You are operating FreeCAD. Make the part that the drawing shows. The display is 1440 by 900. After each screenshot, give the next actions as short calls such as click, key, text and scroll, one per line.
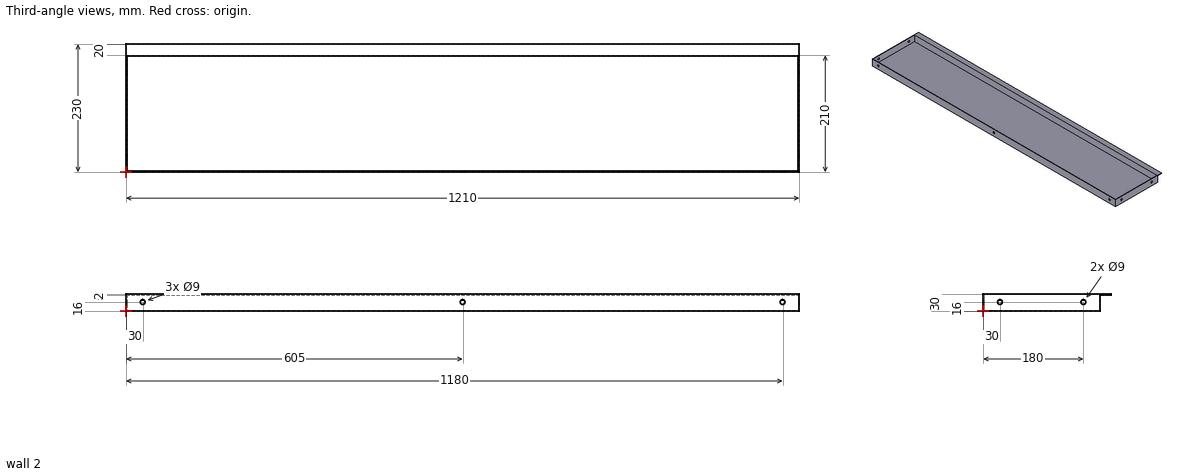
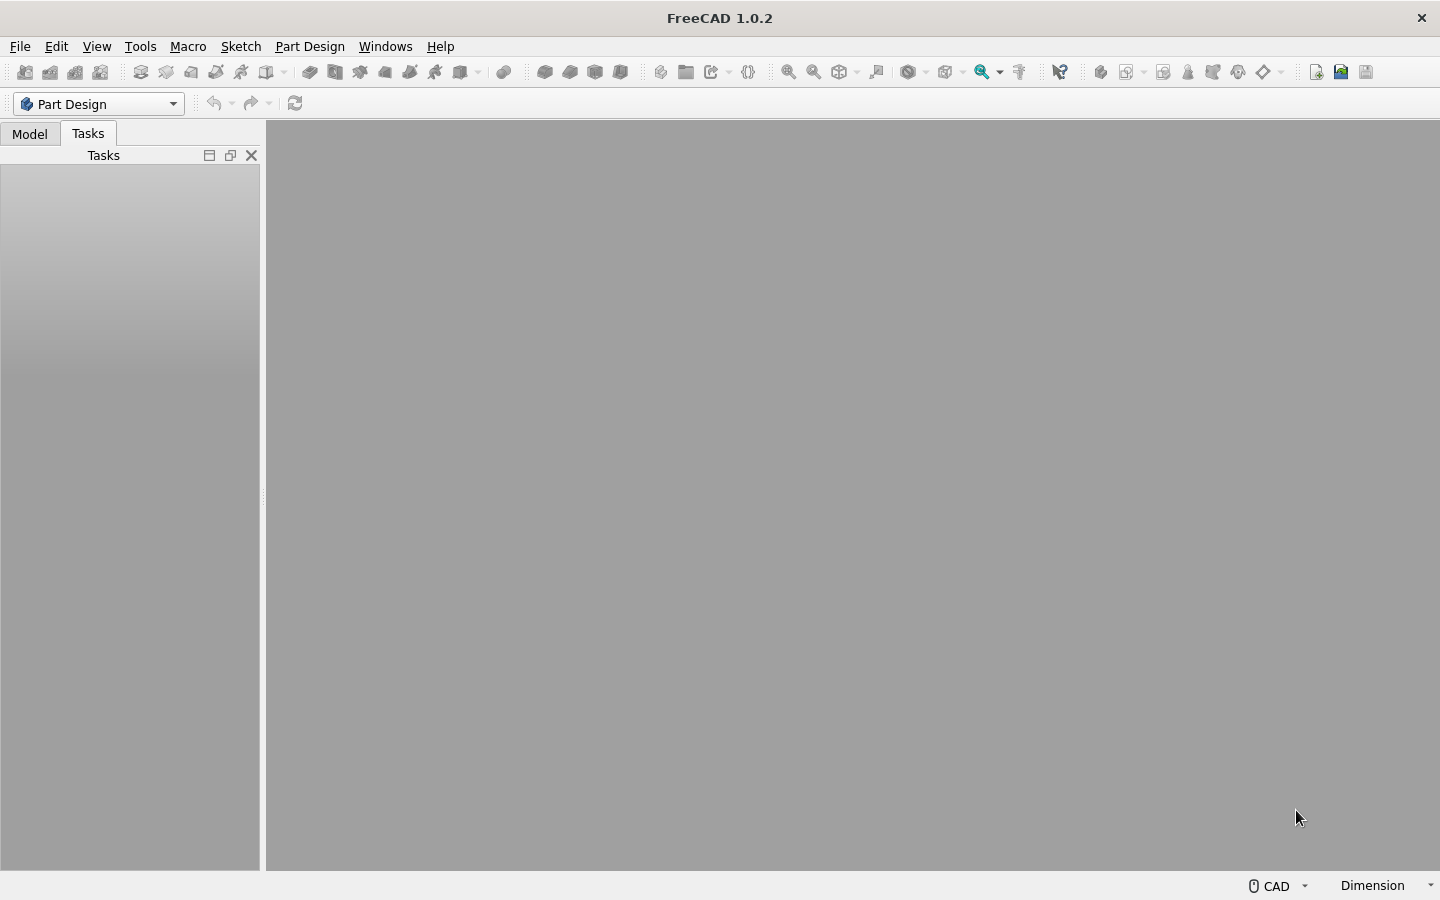
key(ctrl+n)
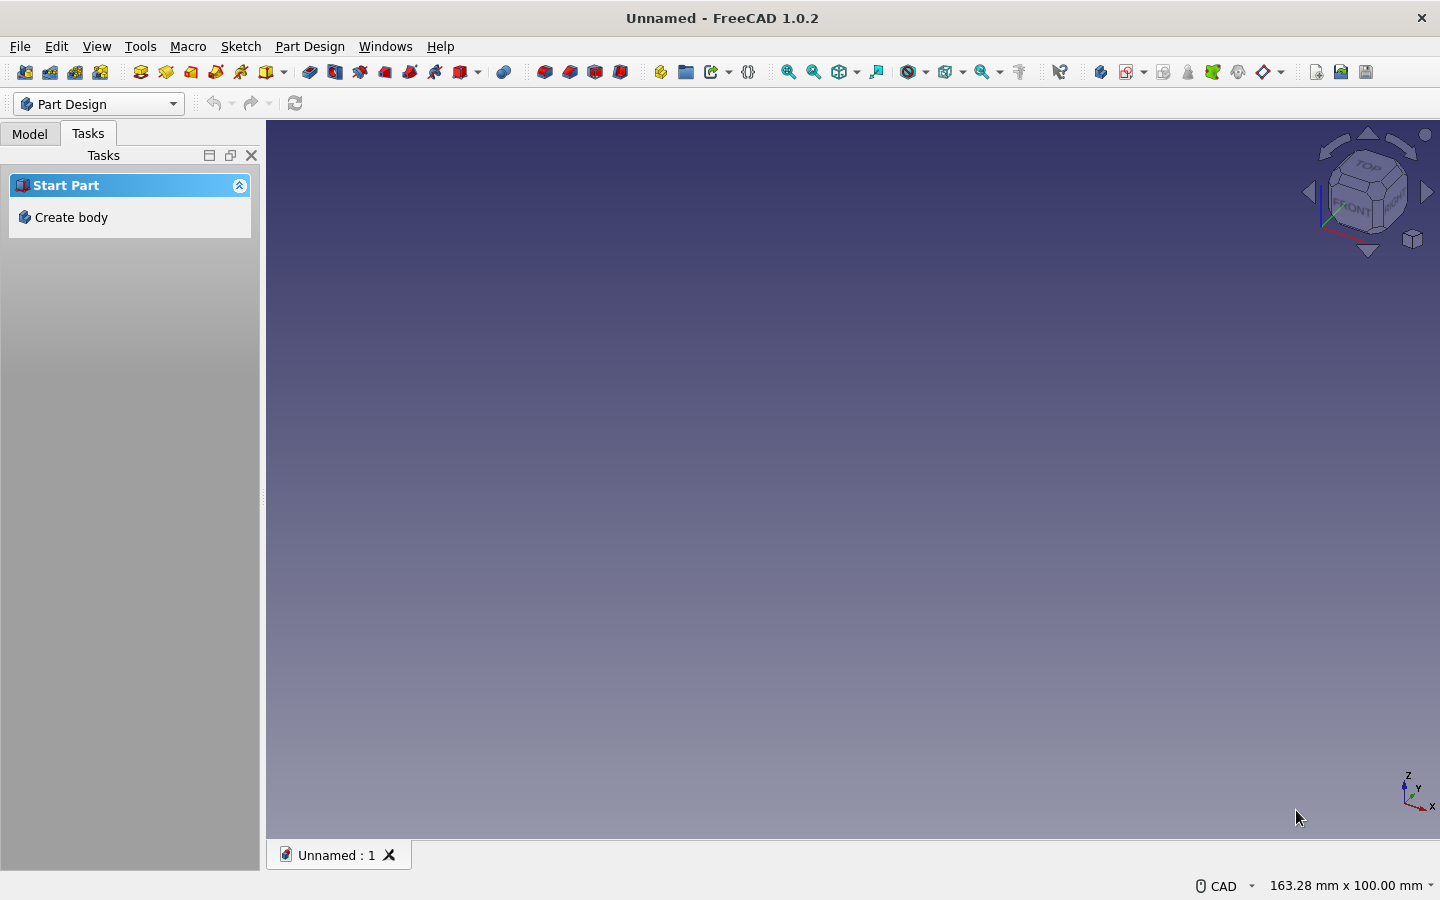
click(1126, 72)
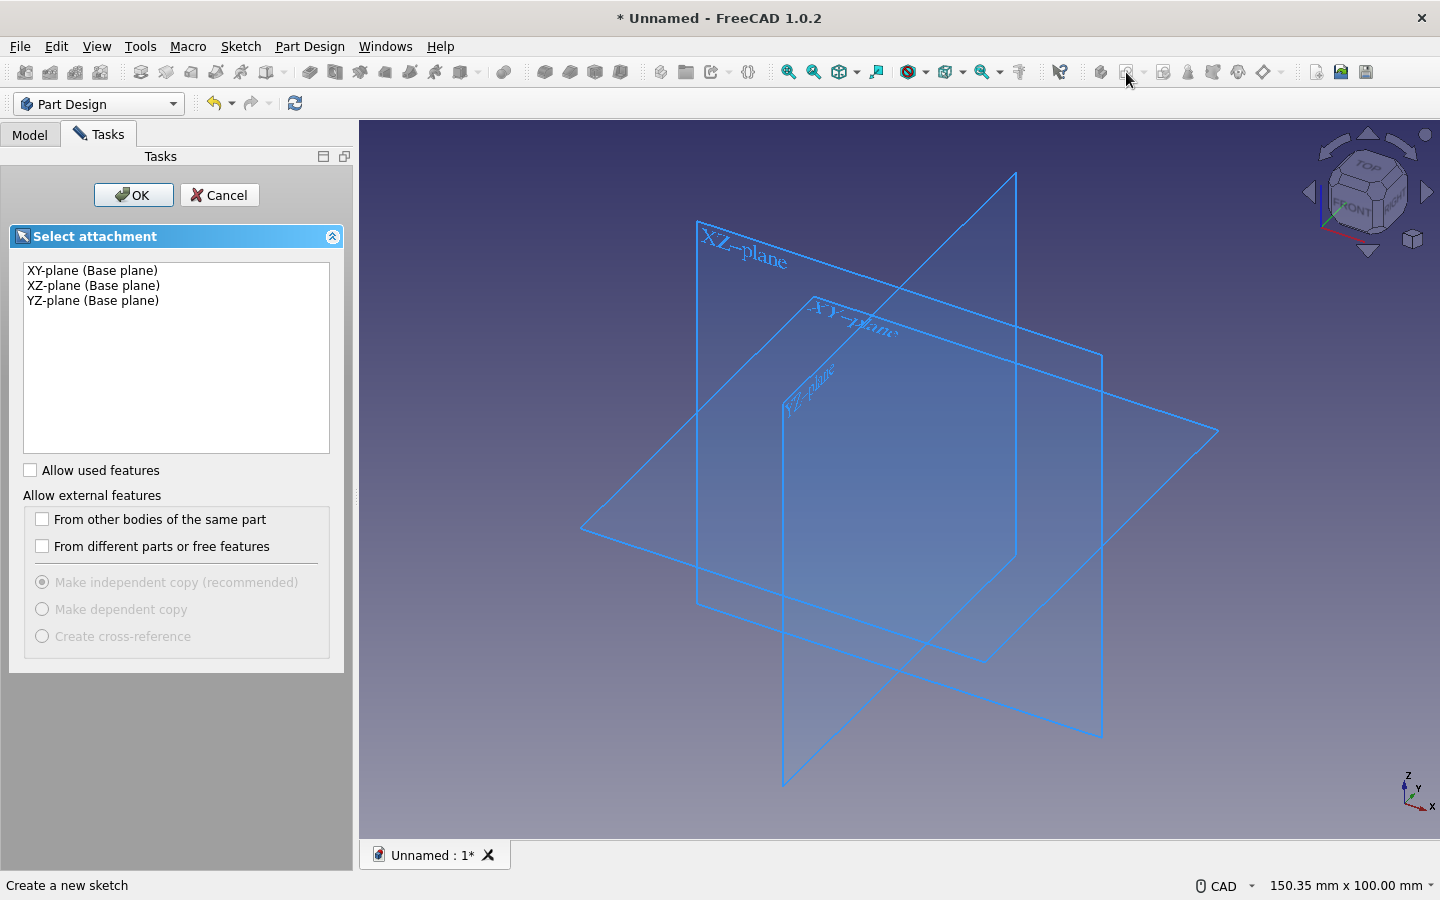
click(84, 270)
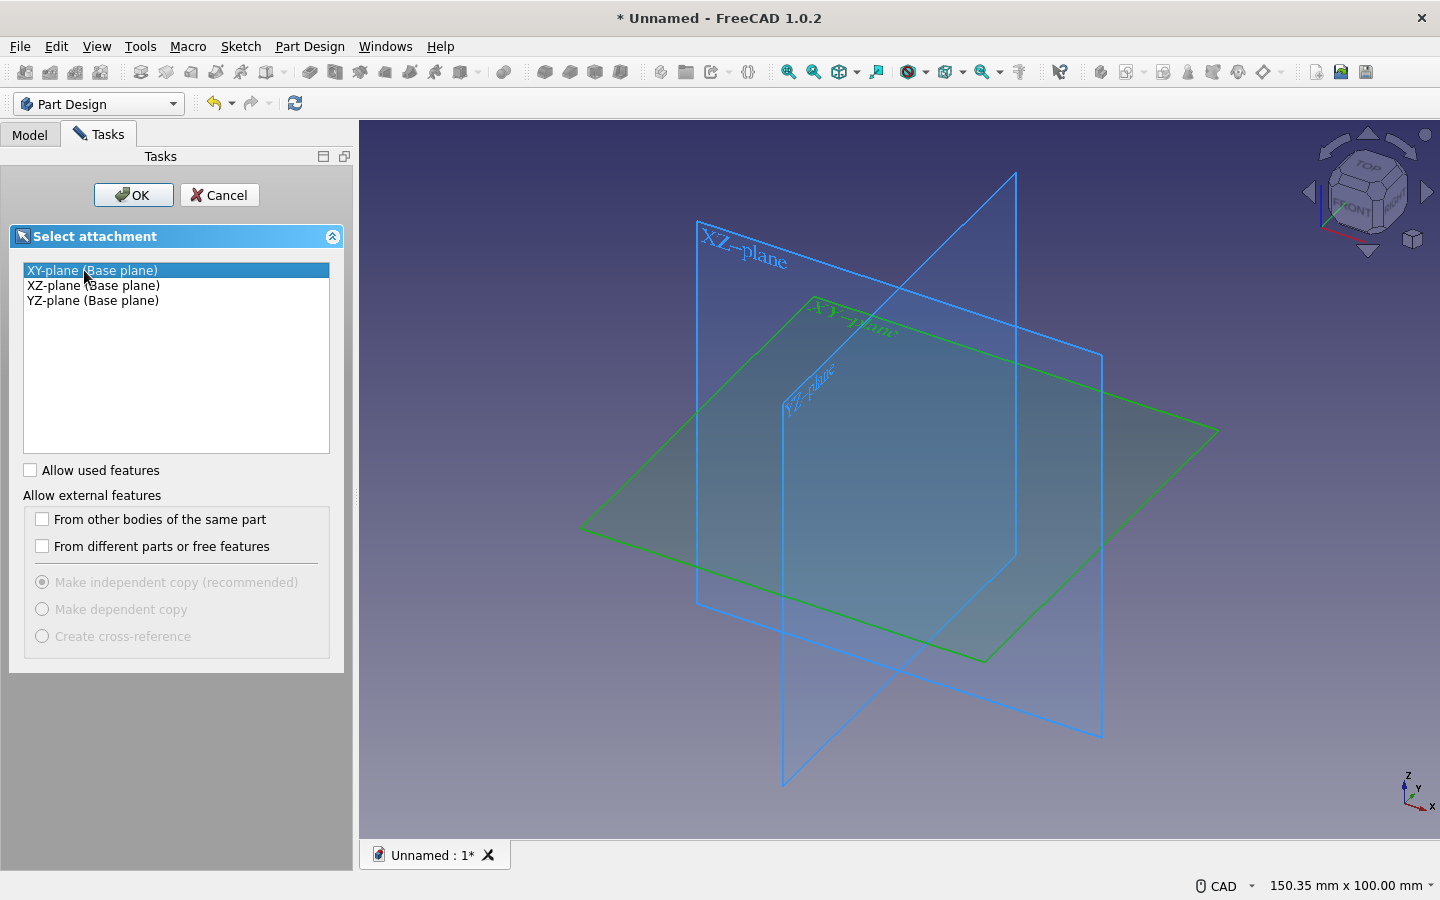
click(134, 195)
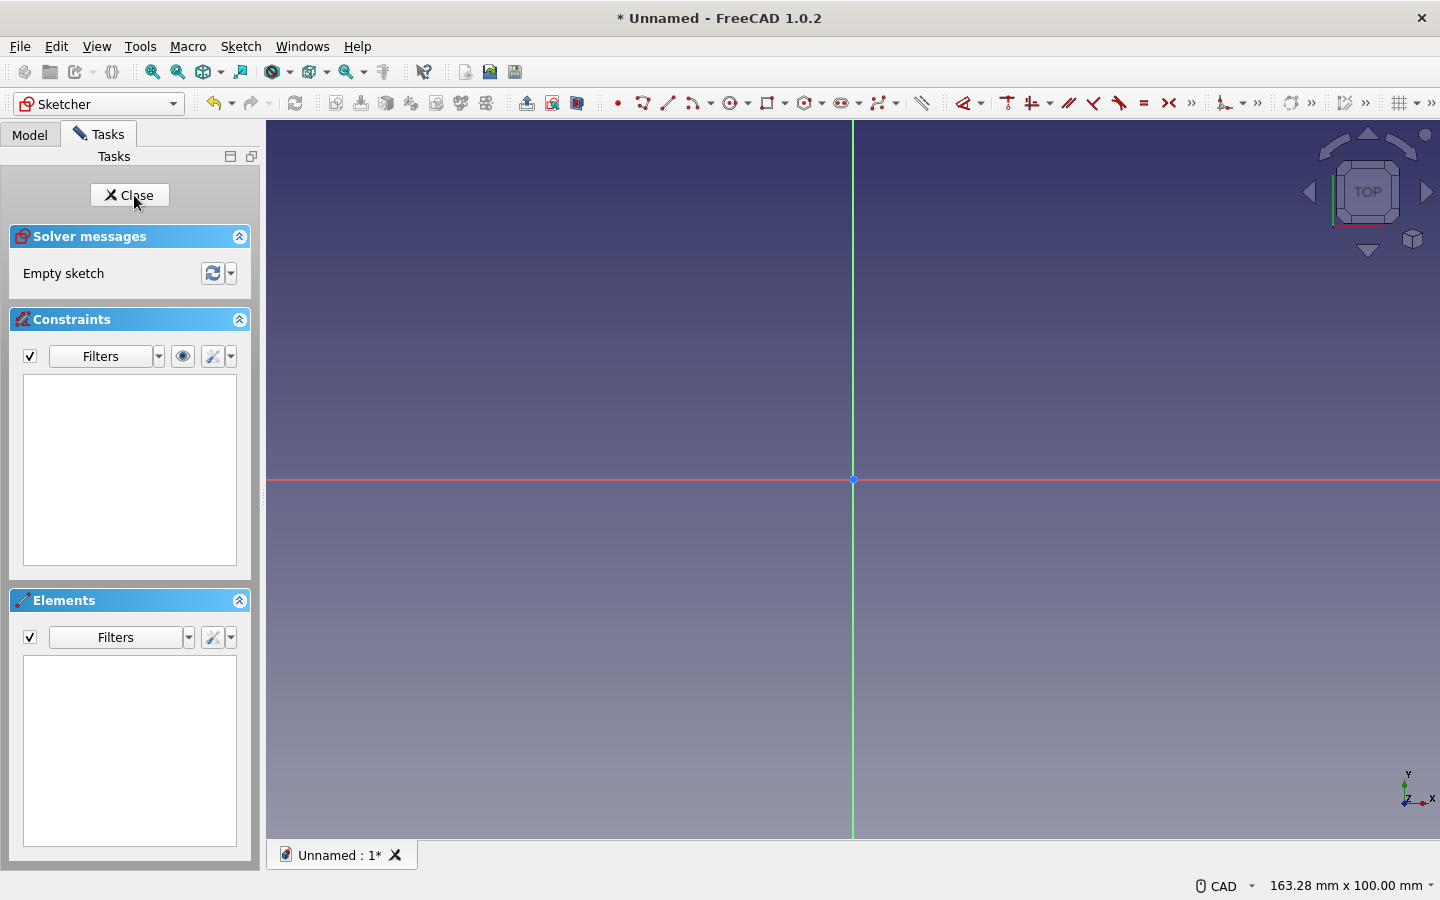
scroll(430, 540, down, 13)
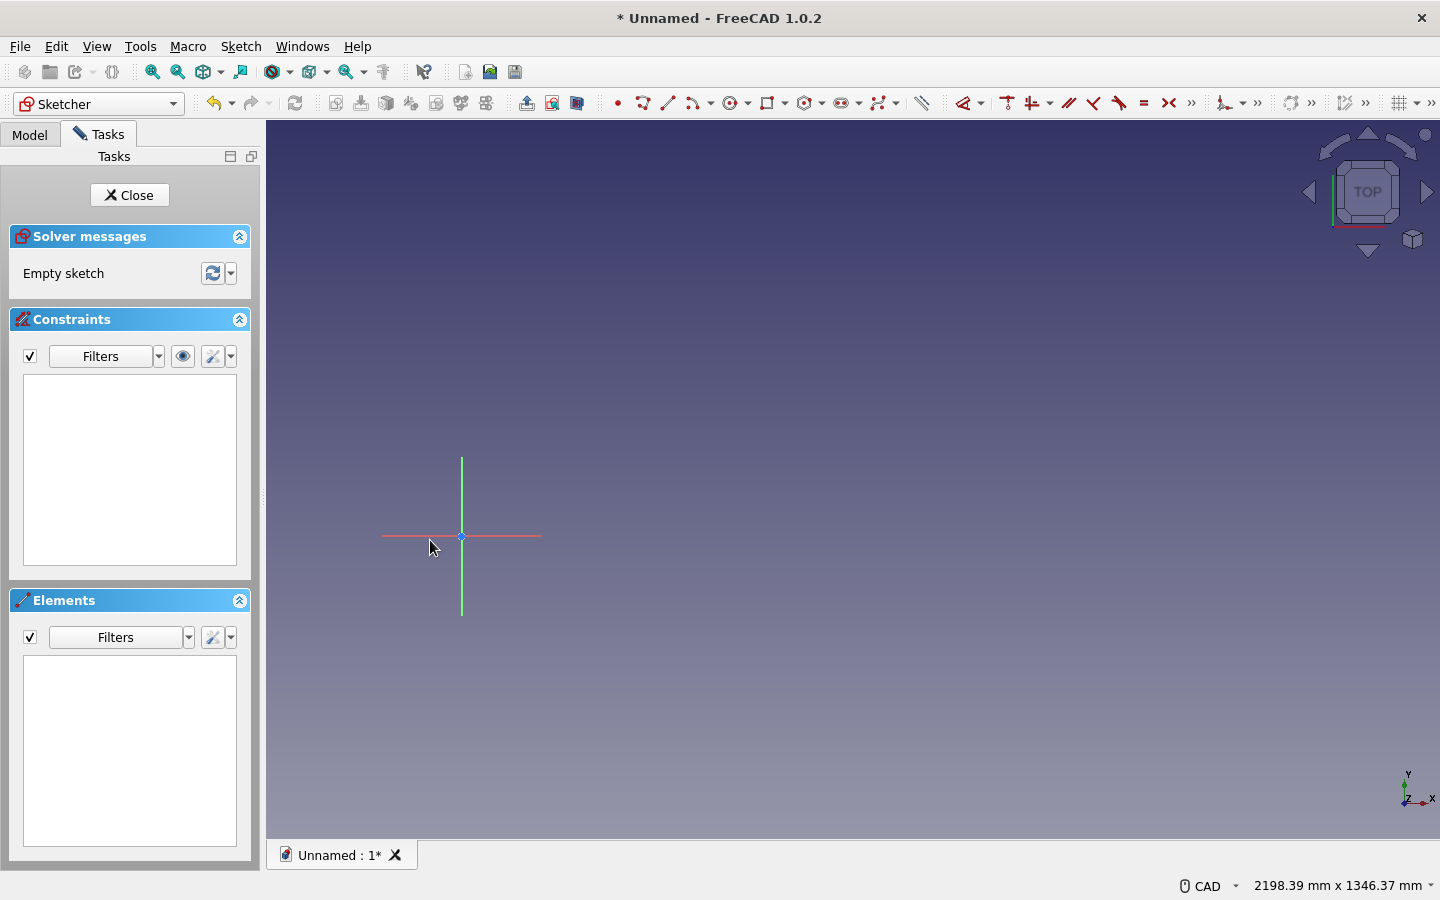
click(766, 104)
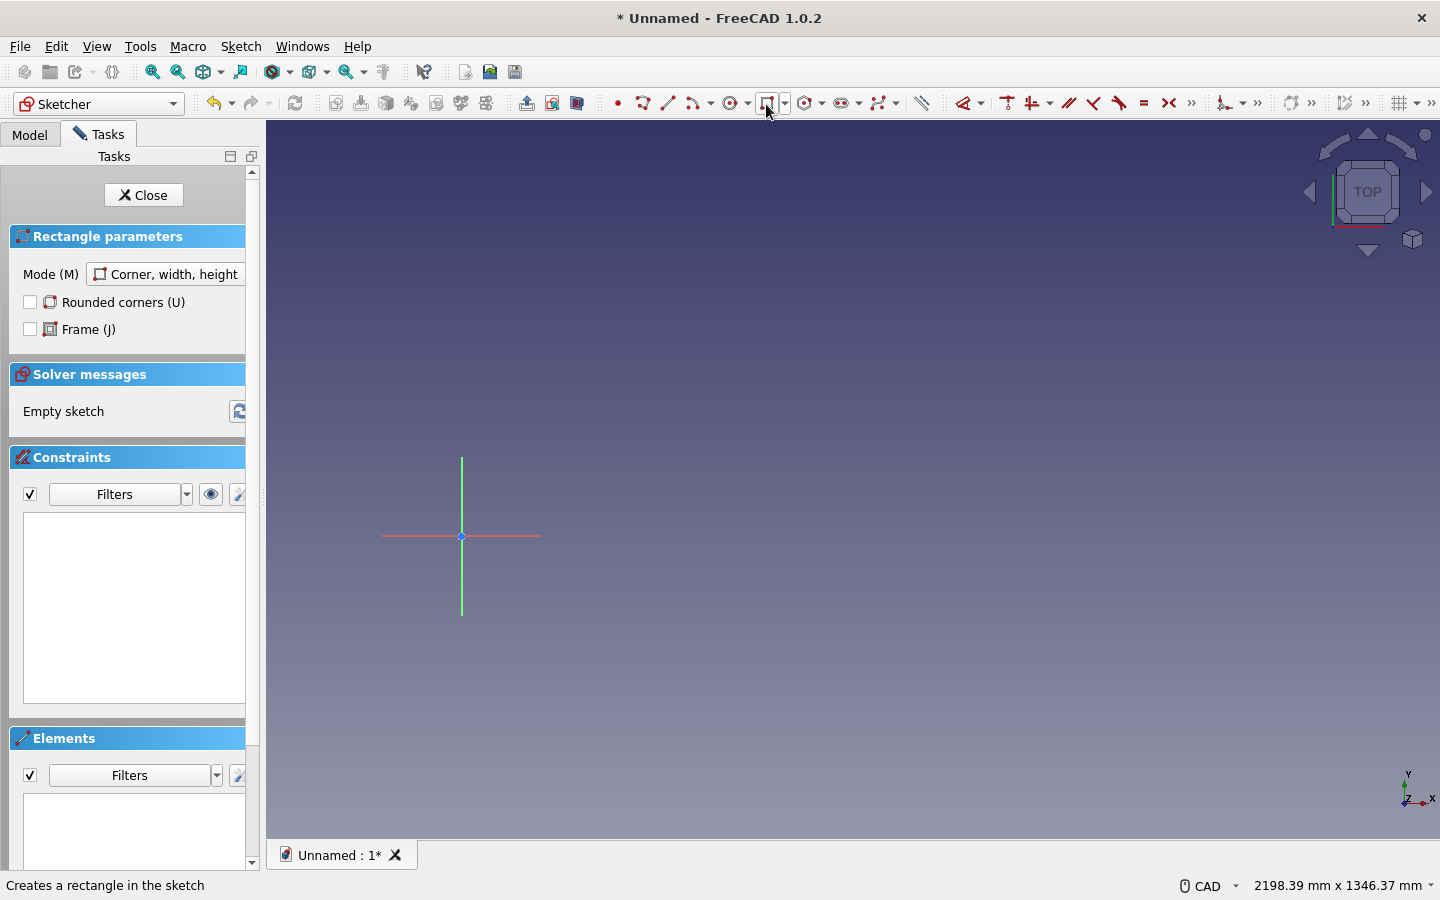
click(462, 536)
click(1108, 424)
key(Escape)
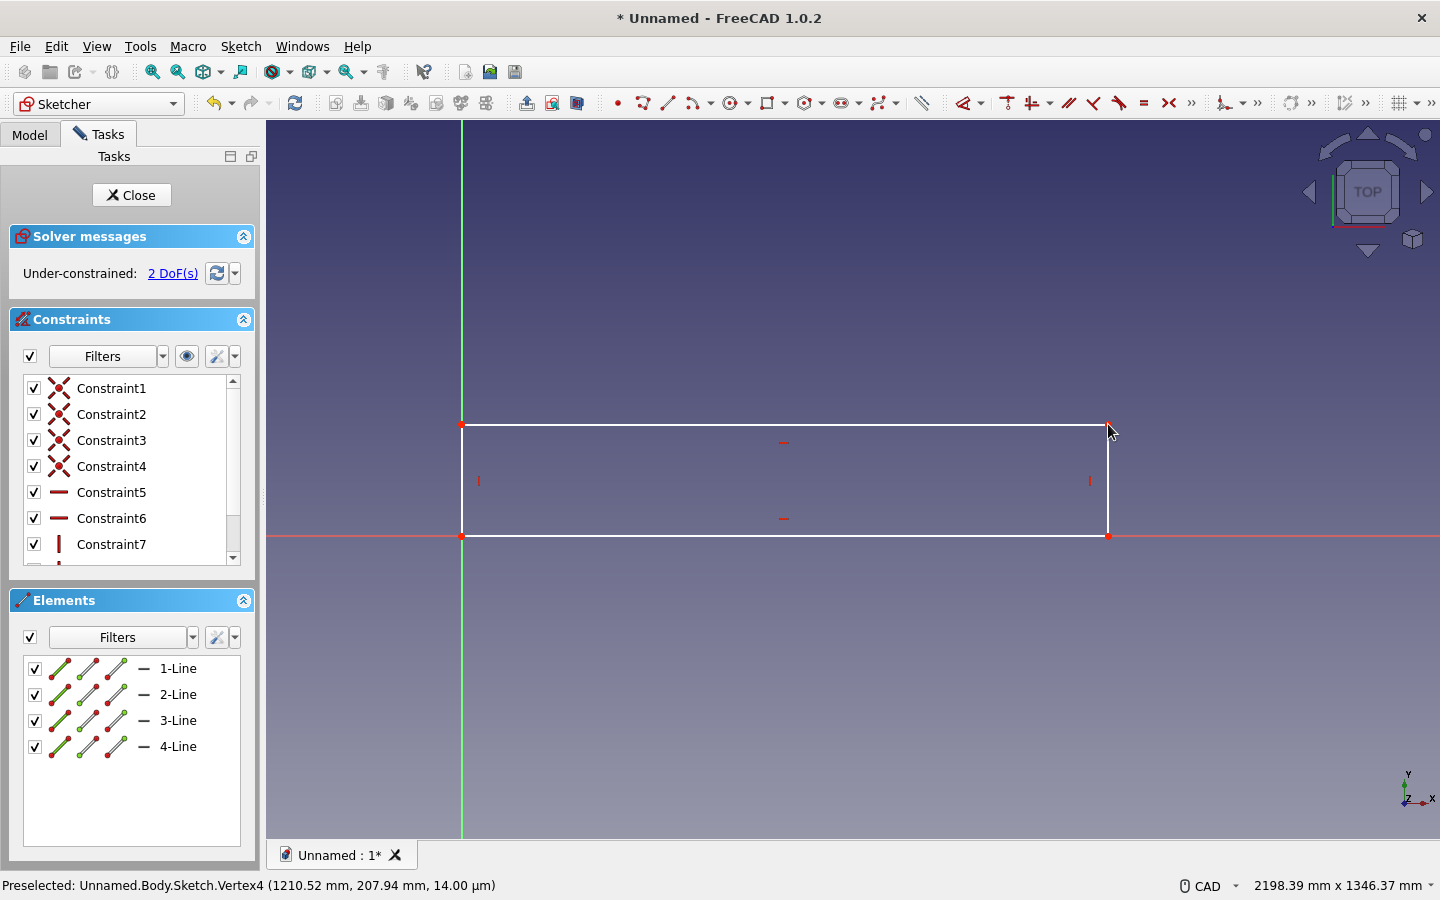
click(962, 104)